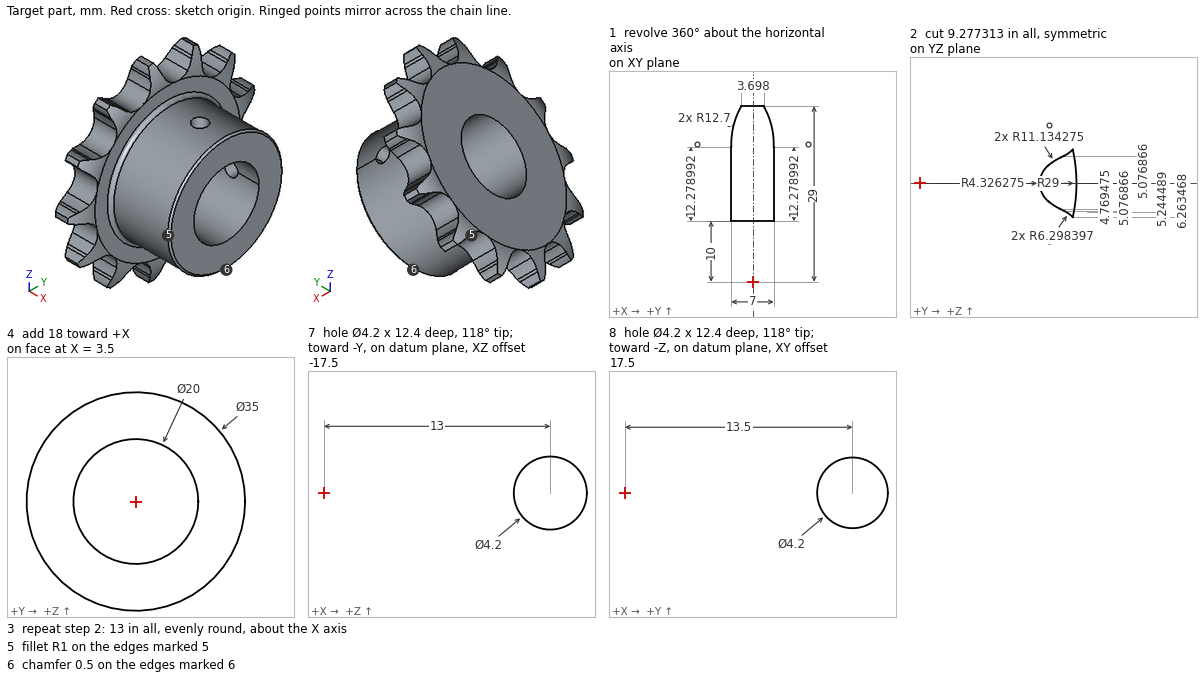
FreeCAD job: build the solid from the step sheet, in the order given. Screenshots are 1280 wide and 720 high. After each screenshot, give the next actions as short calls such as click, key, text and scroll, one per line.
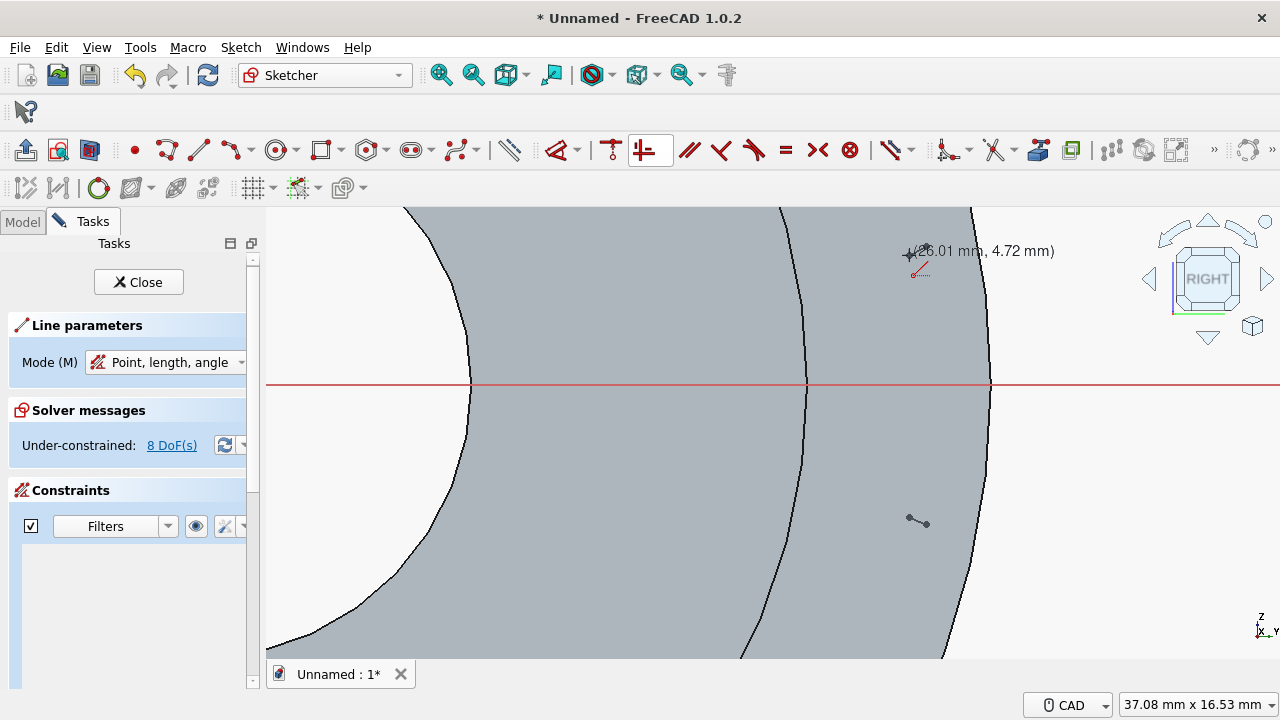
click(232, 150)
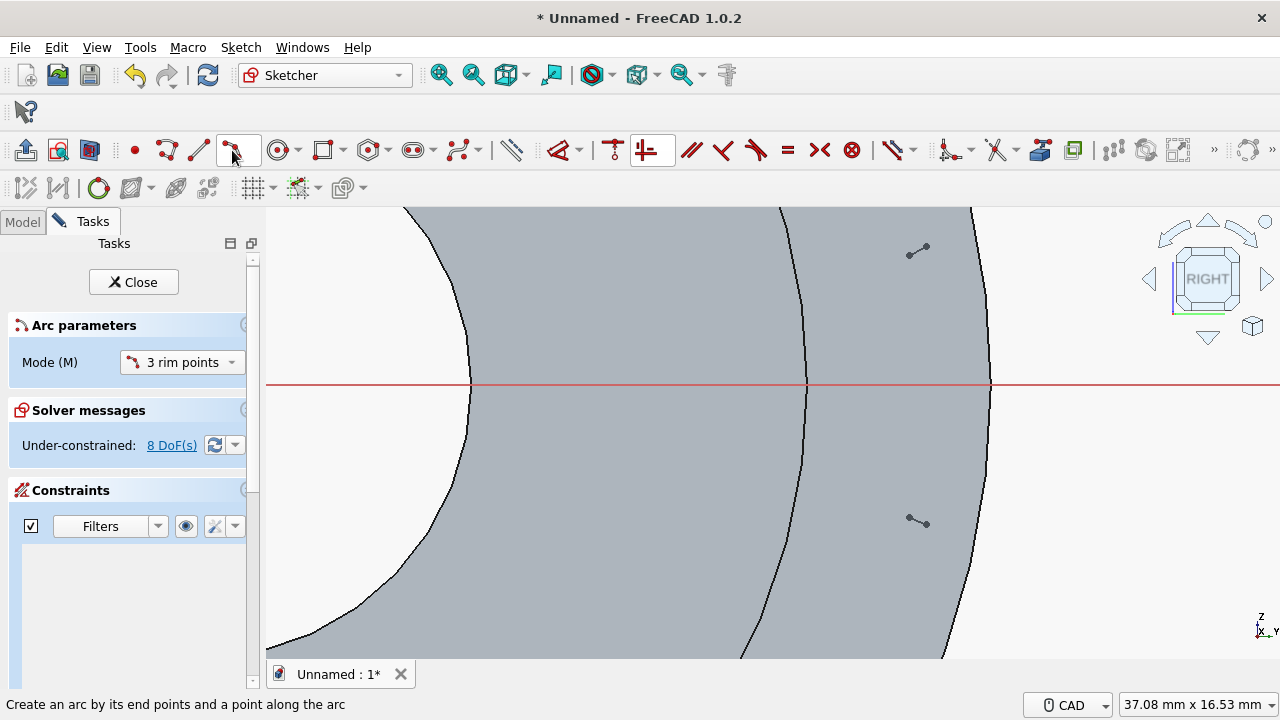
scroll(926, 524, up, 3)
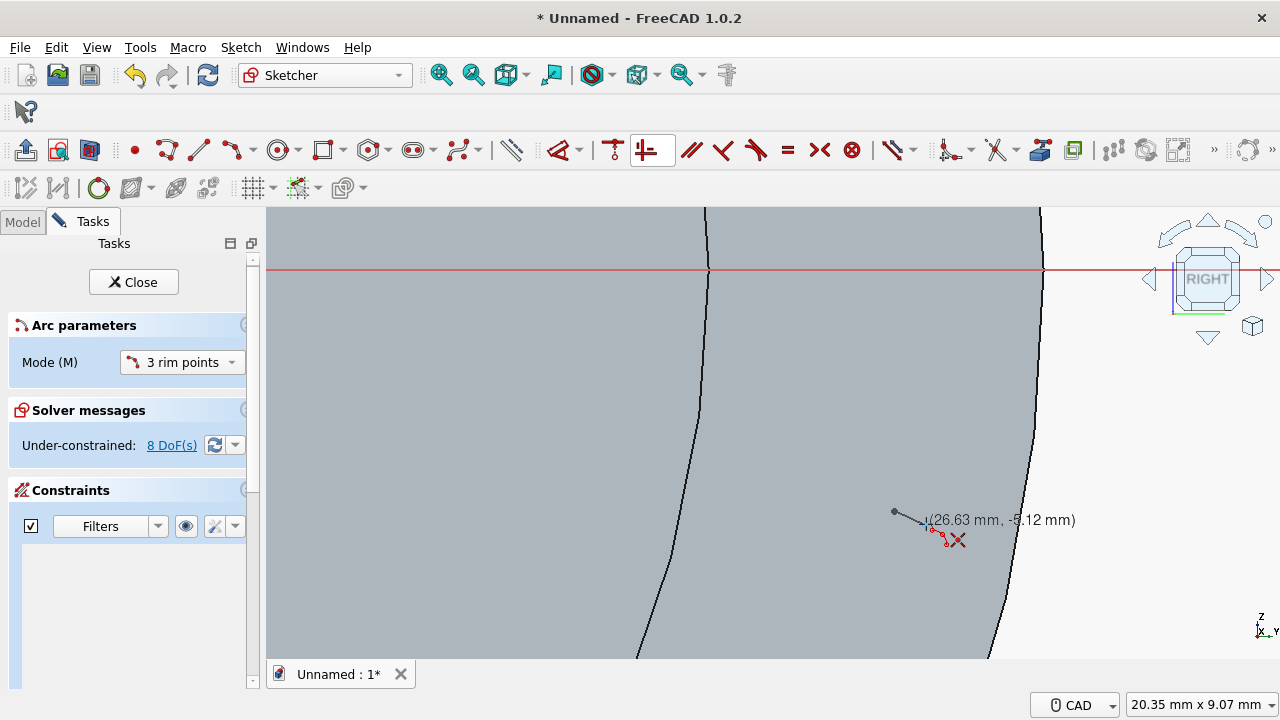
click(925, 525)
click(1010, 582)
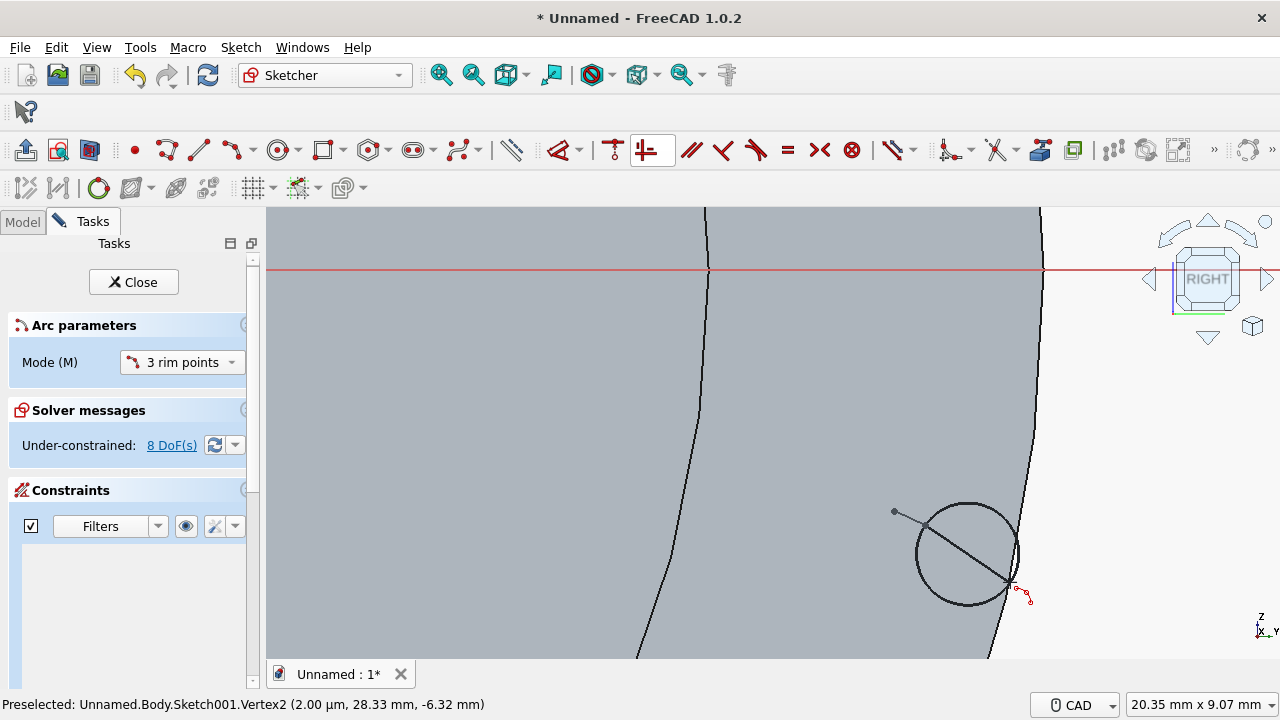
scroll(970, 549, up, 7)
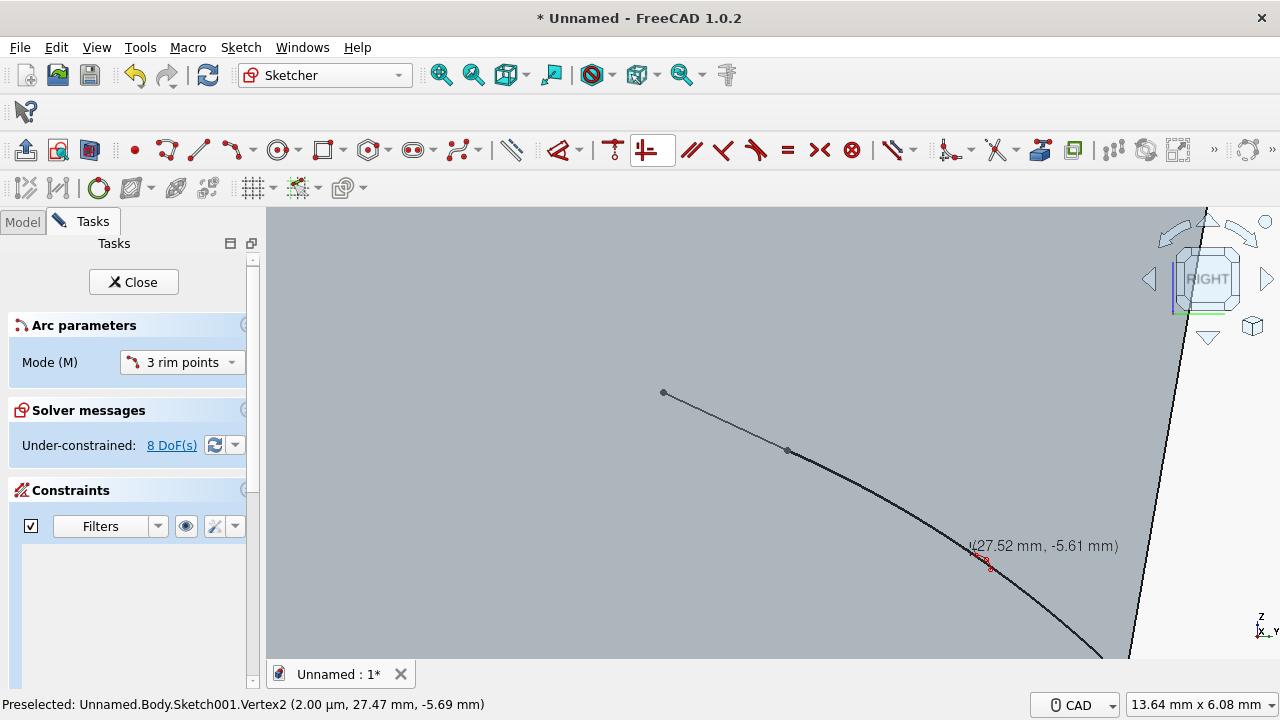
click(969, 549)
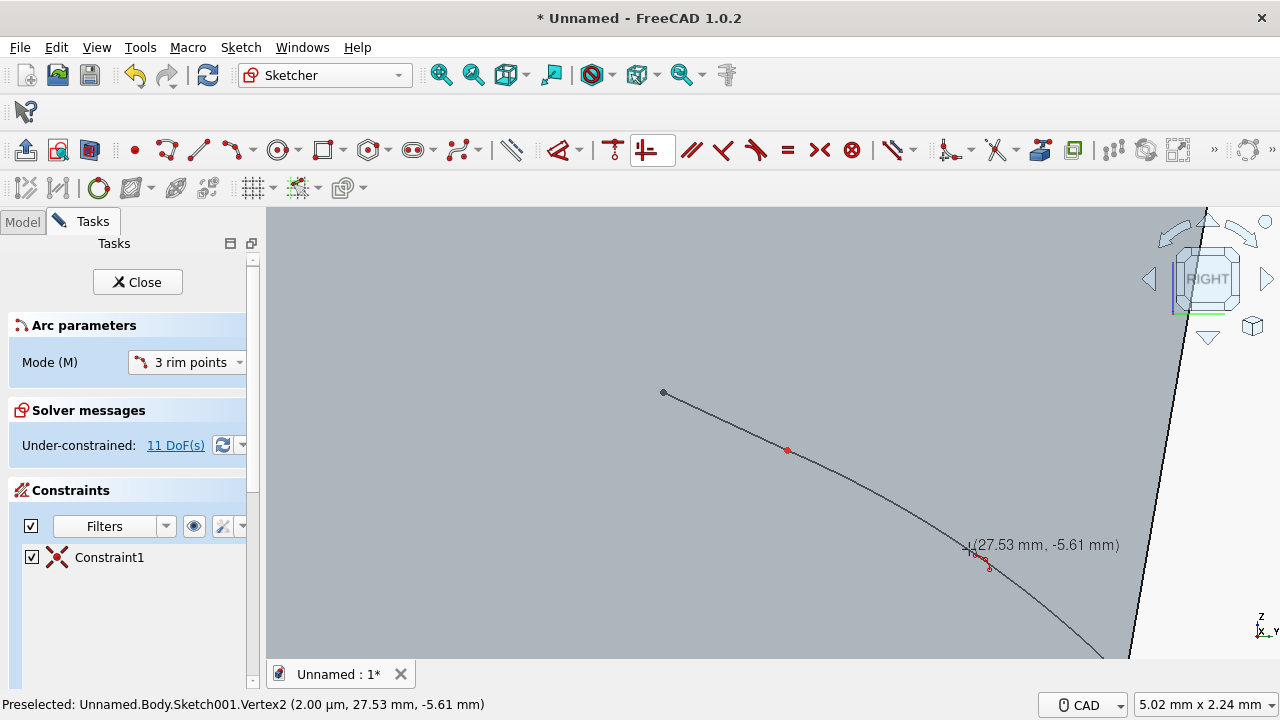
scroll(941, 534, down, 12)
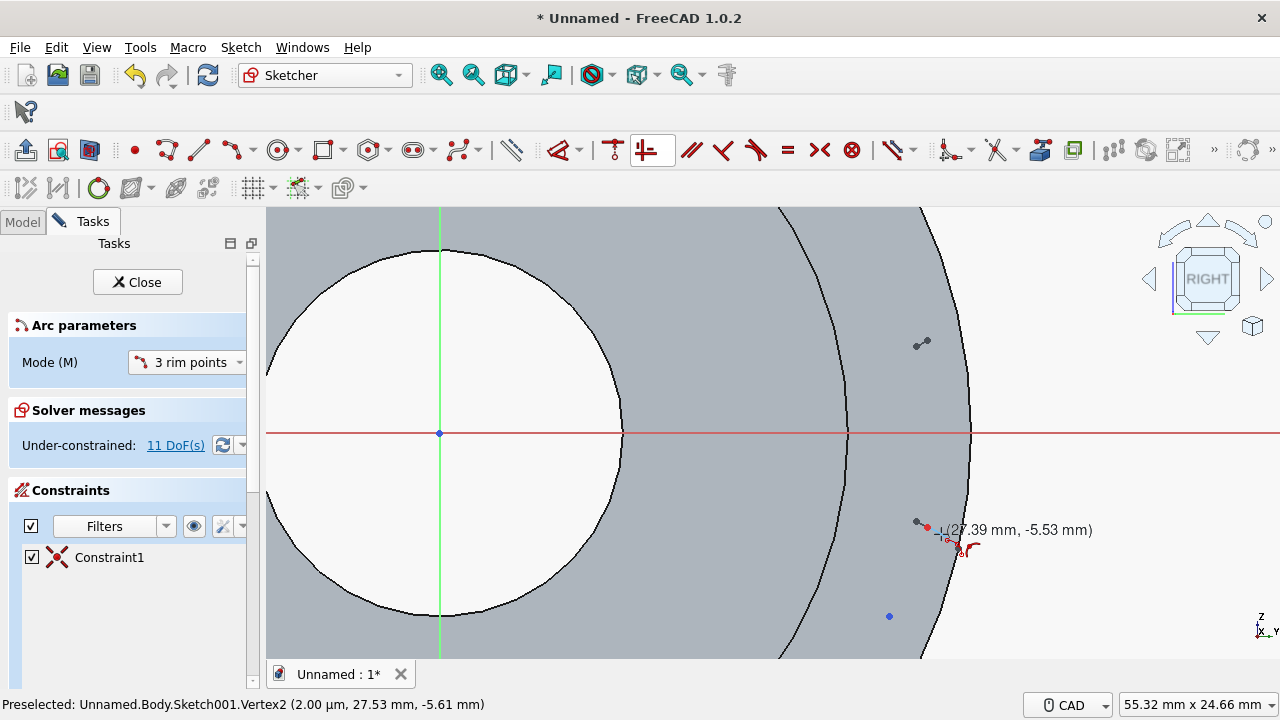
click(959, 548)
click(959, 319)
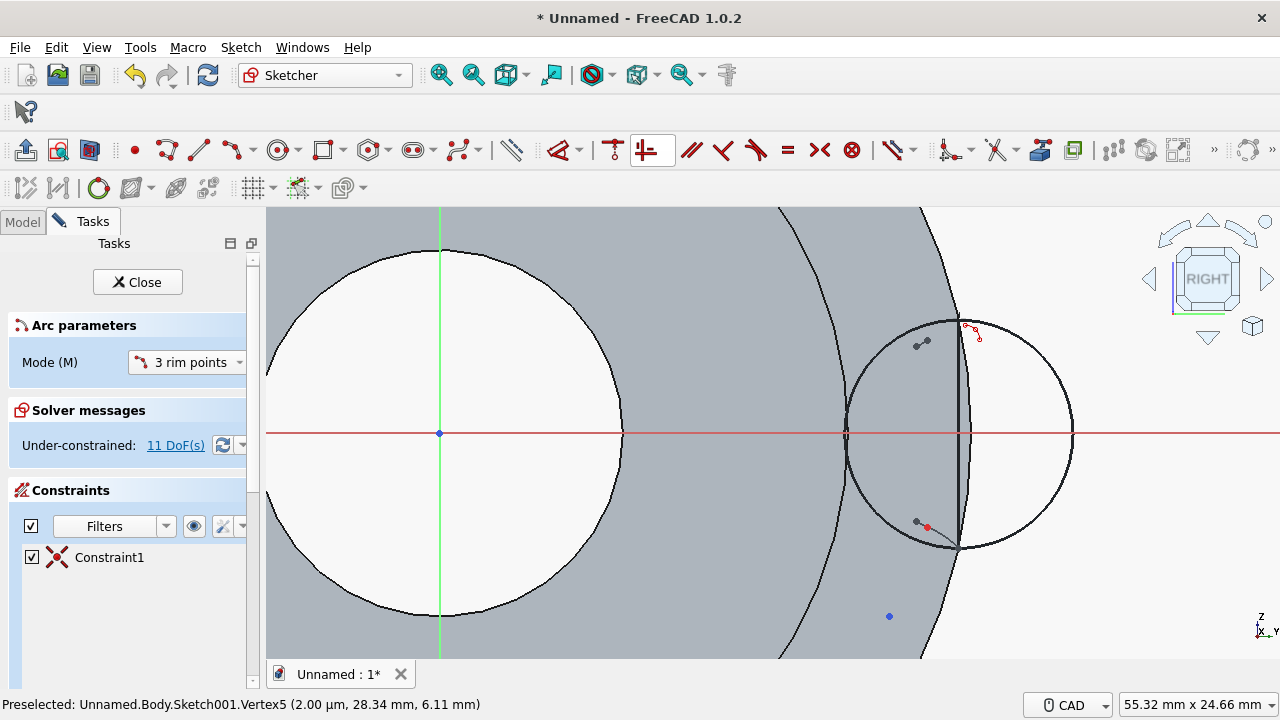
scroll(971, 456, up, 2)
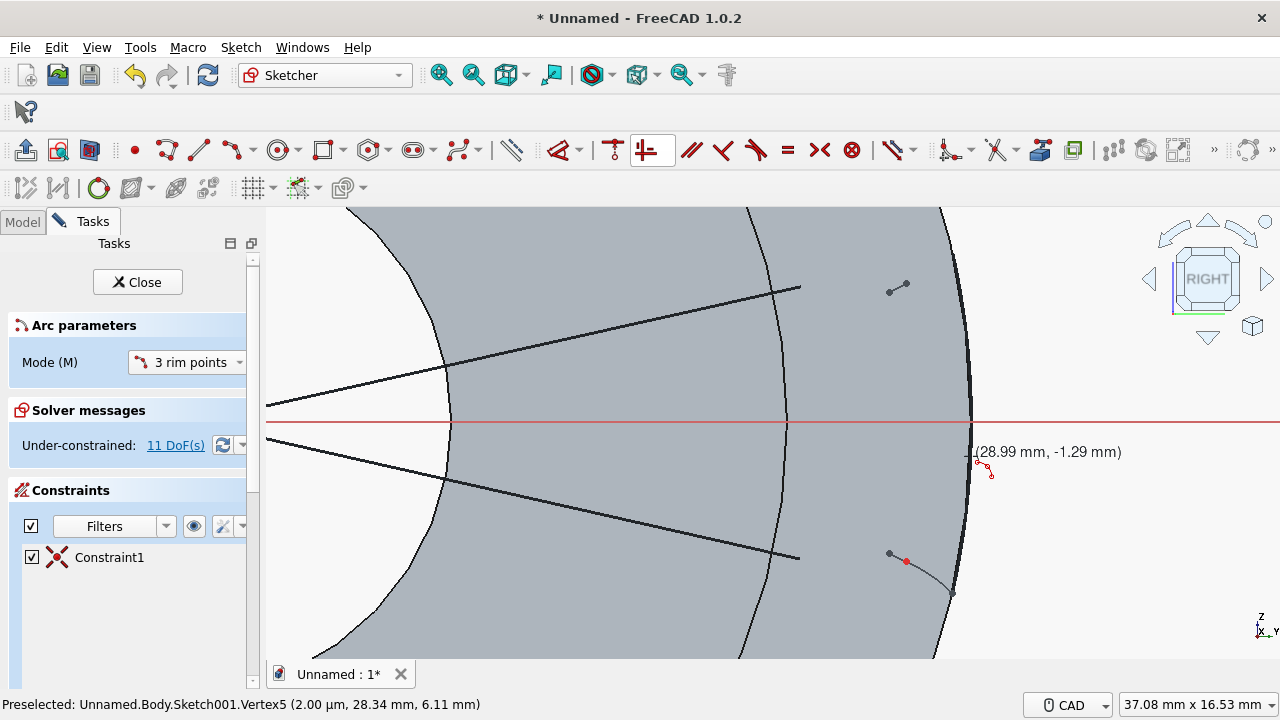
click(970, 456)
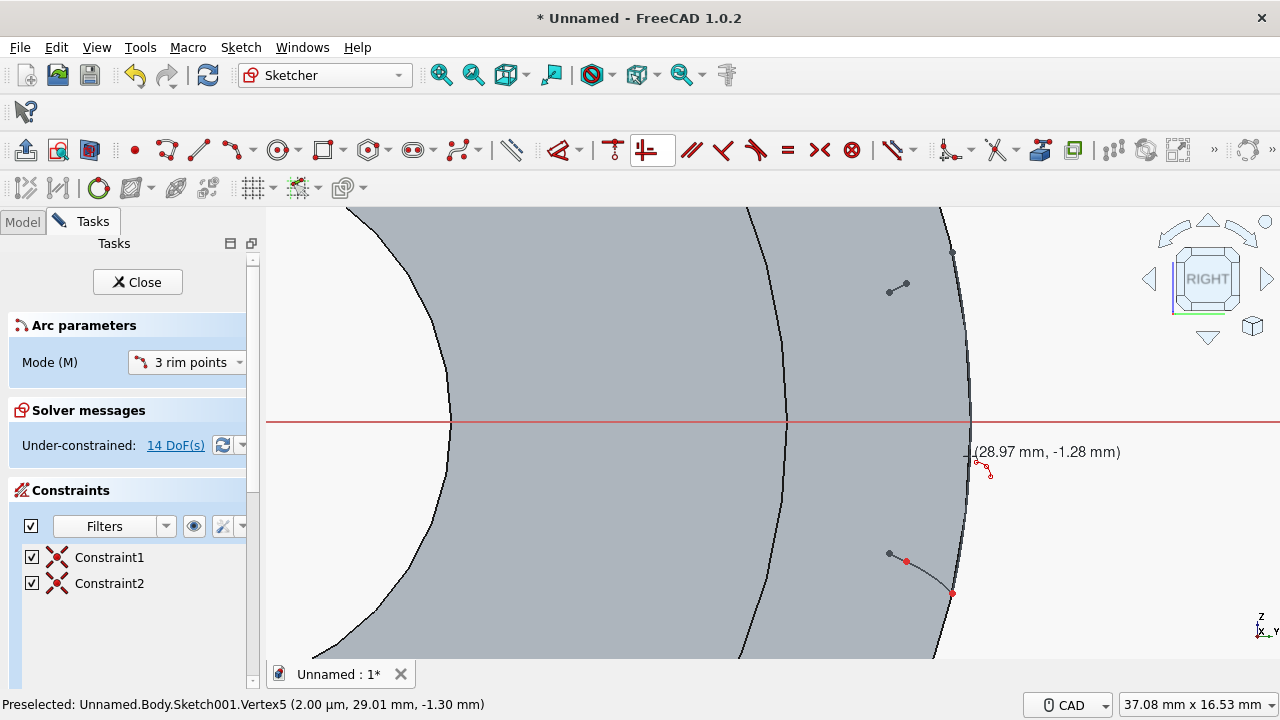
click(953, 253)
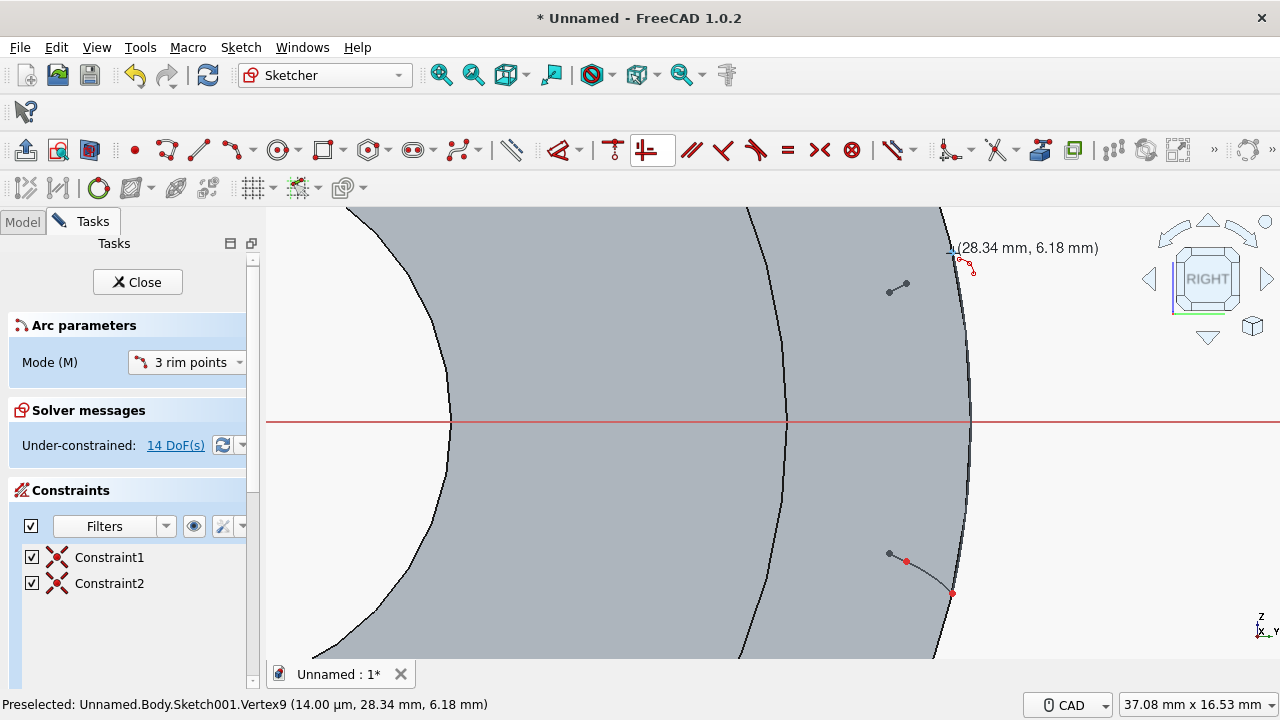
scroll(906, 283, up, 3)